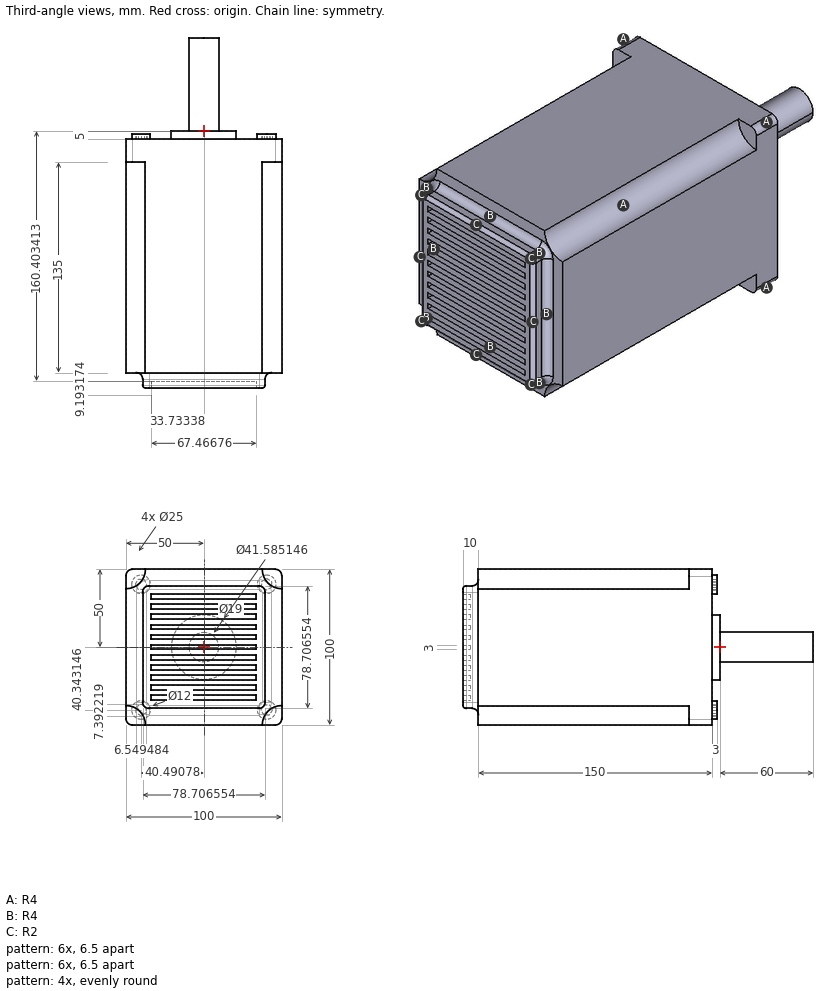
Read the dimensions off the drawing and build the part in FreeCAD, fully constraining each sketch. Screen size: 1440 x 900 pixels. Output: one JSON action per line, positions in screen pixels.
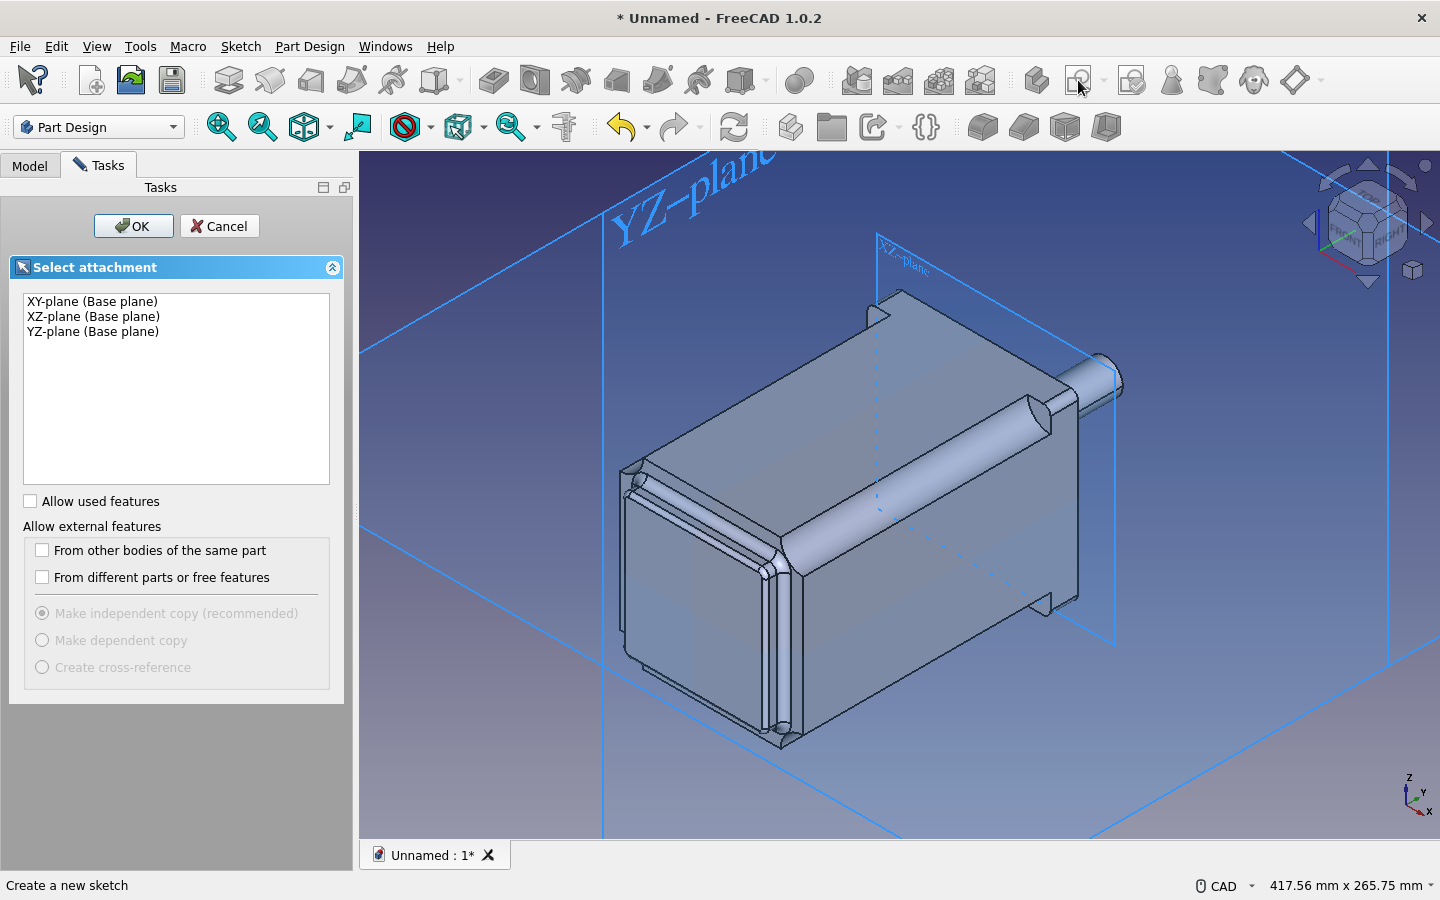
{"action": "left_click", "coordinate": [84, 302]}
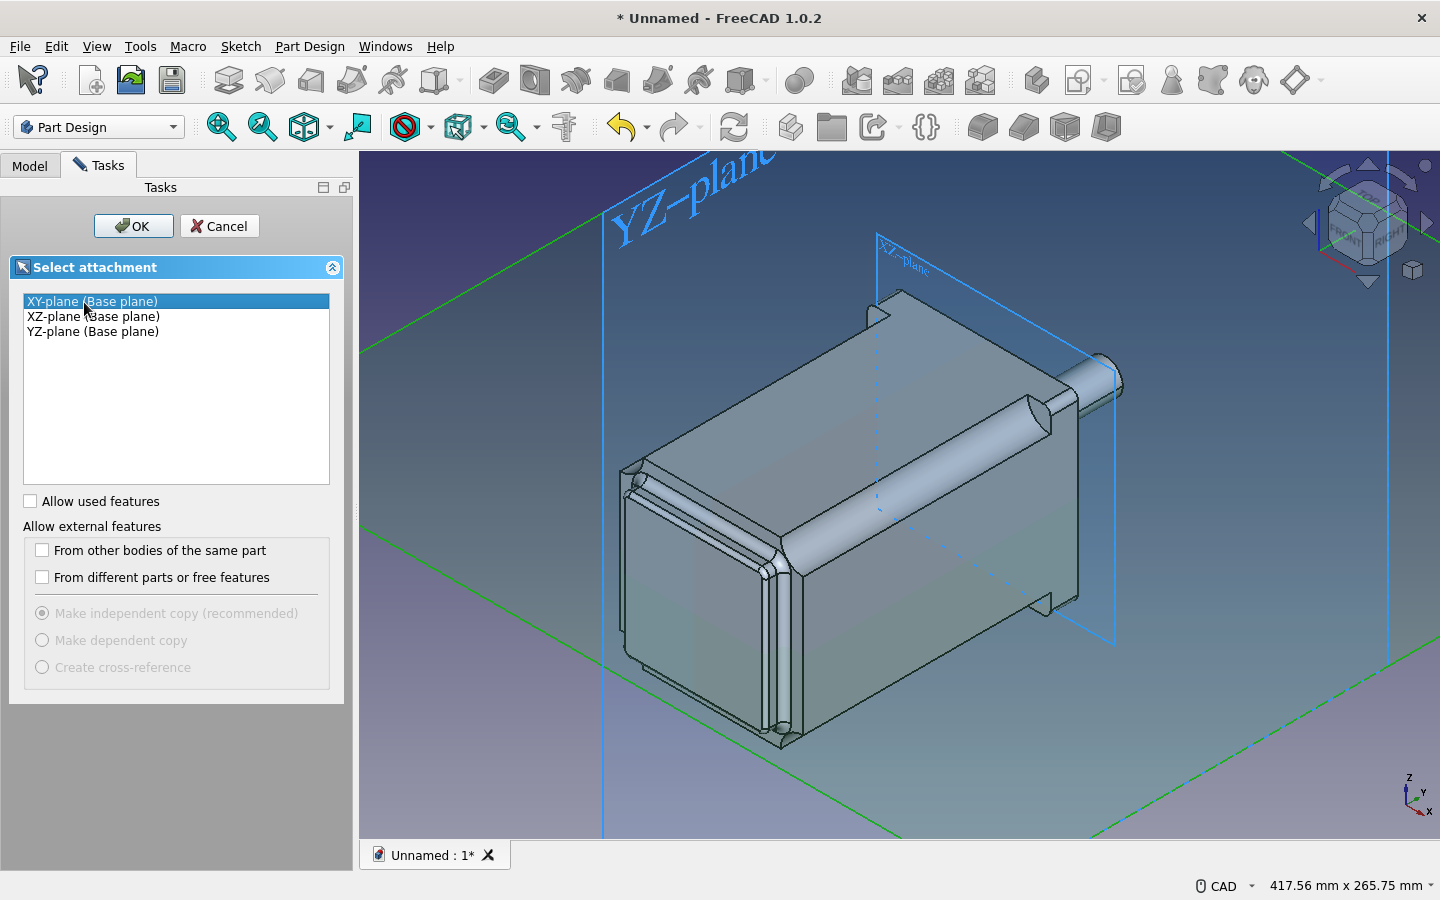
{"action": "left_click", "coordinate": [134, 226]}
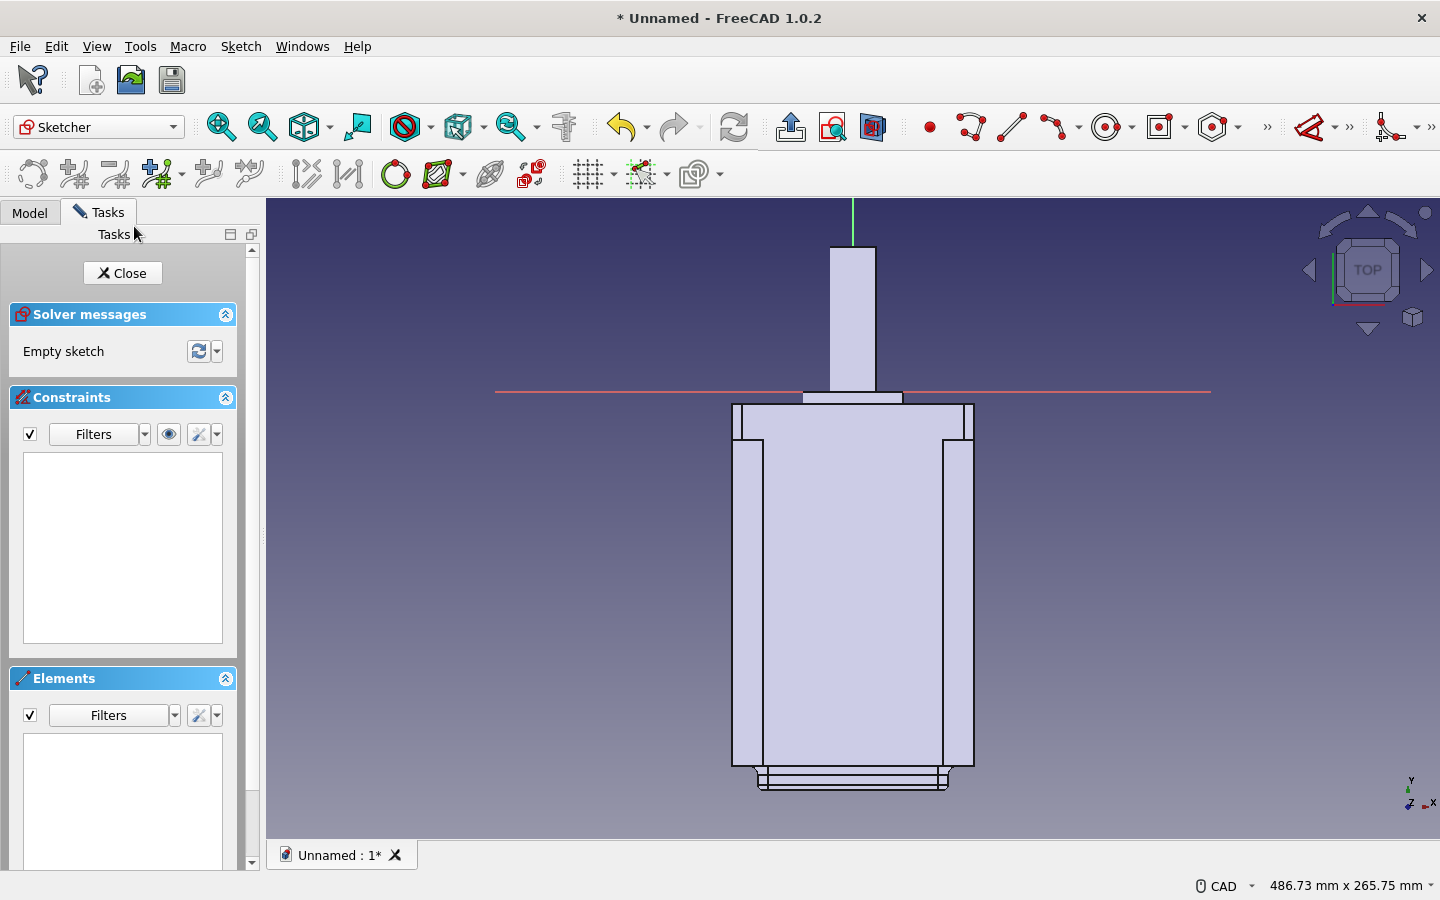
{"action": "left_click", "coordinate": [873, 128]}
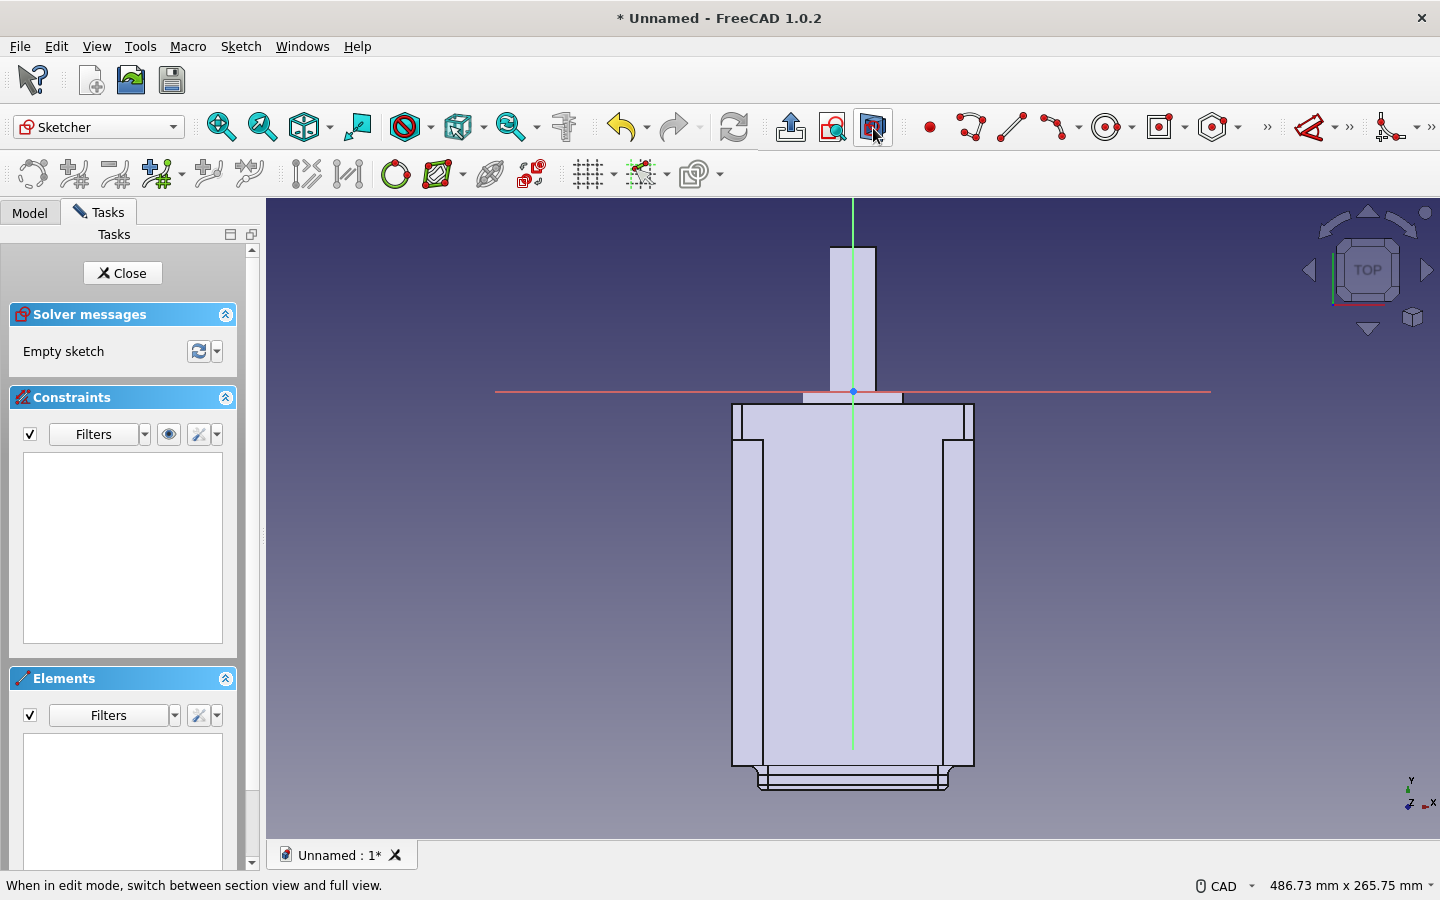
{"action": "scroll", "coordinate": [875, 811], "scroll_direction": "up", "scroll_amount": 7}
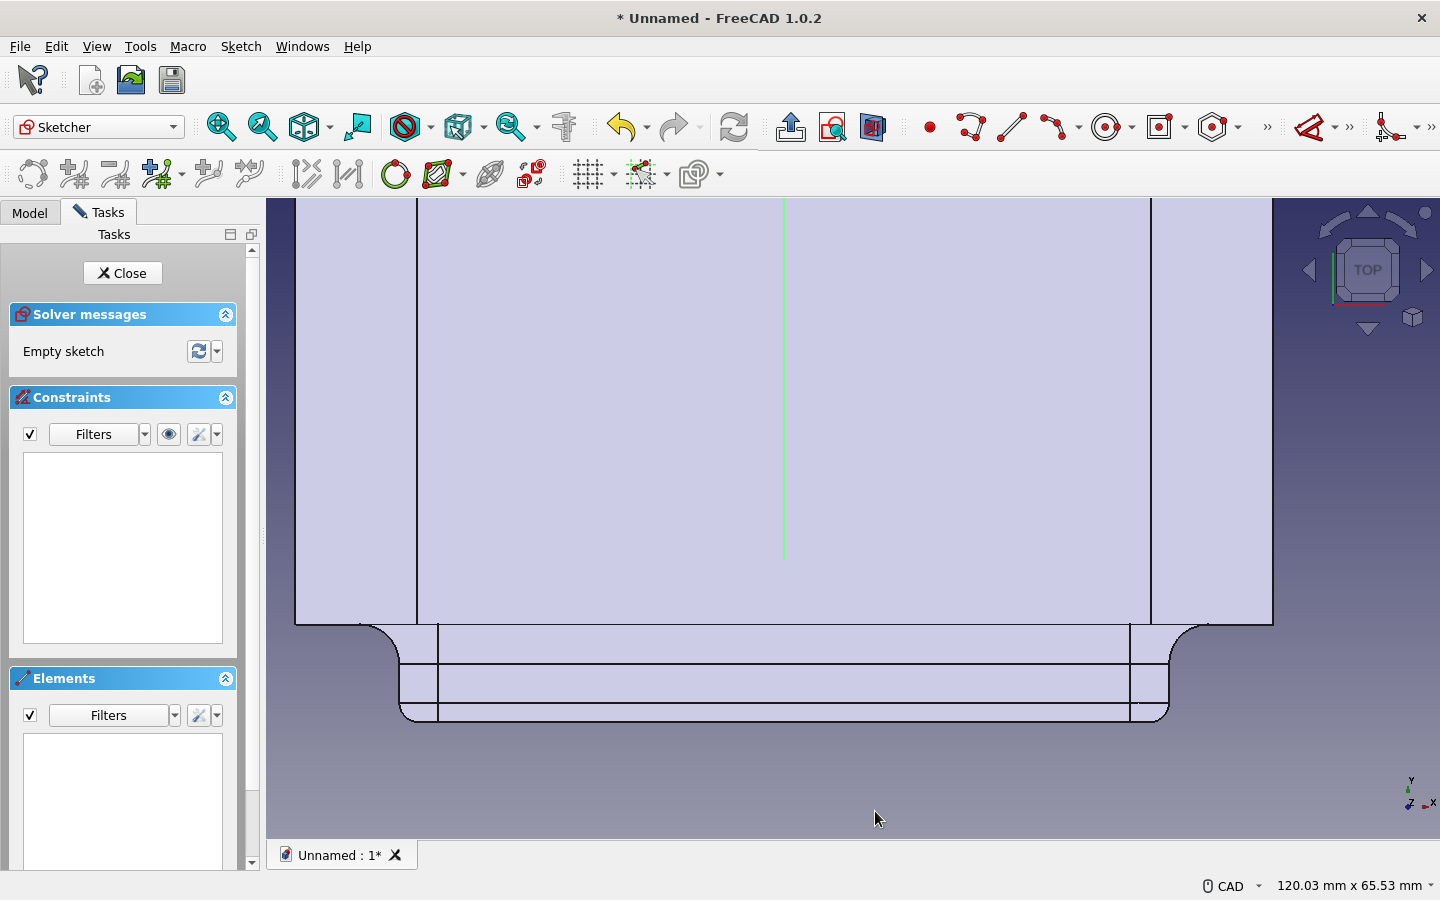
{"action": "left_click", "coordinate": [1184, 128]}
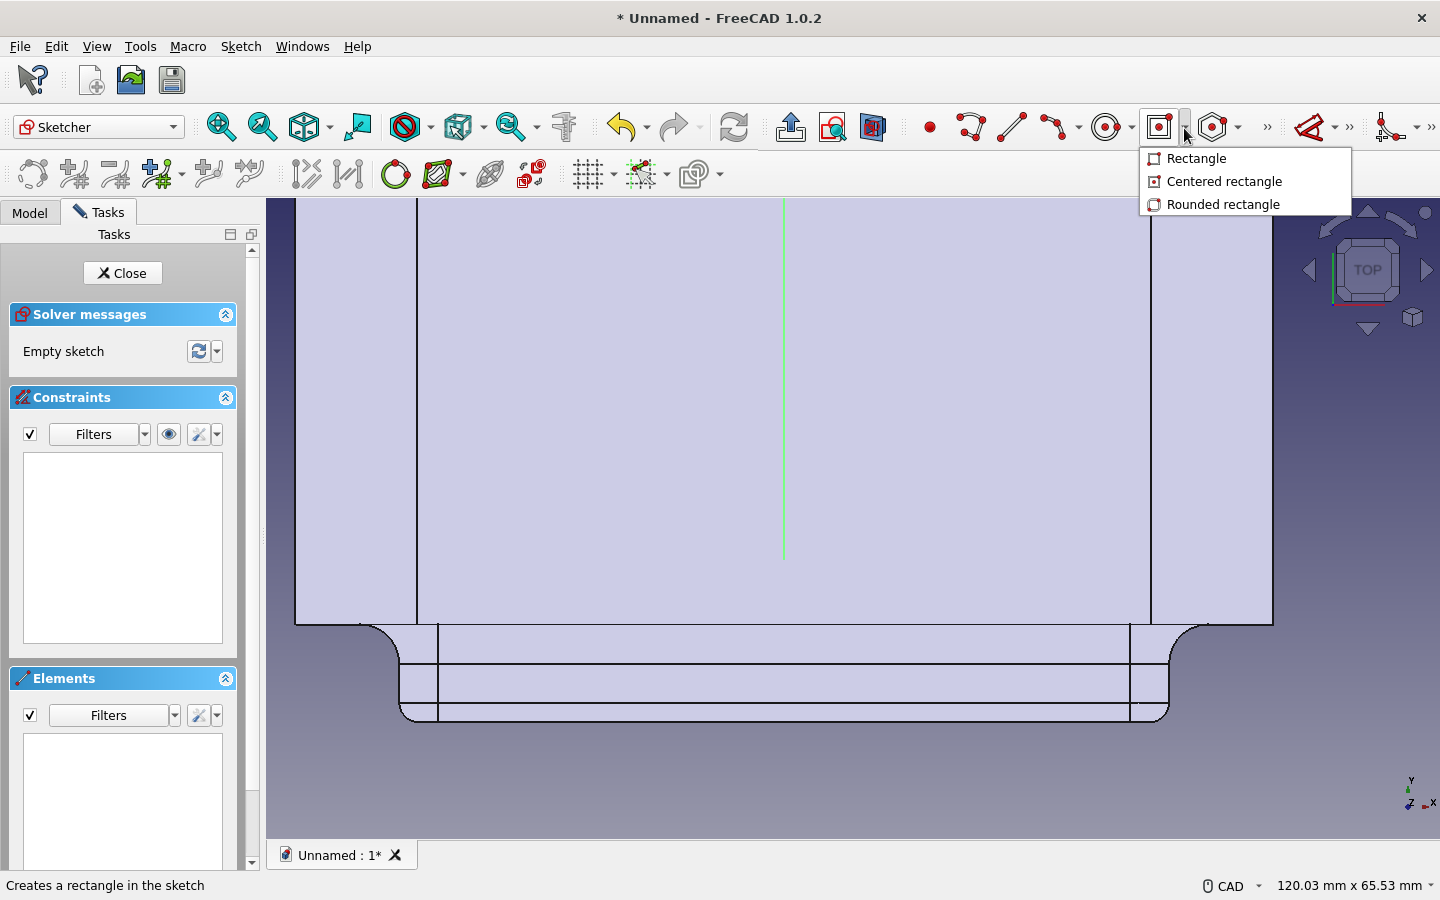
{"action": "left_click", "coordinate": [1246, 158]}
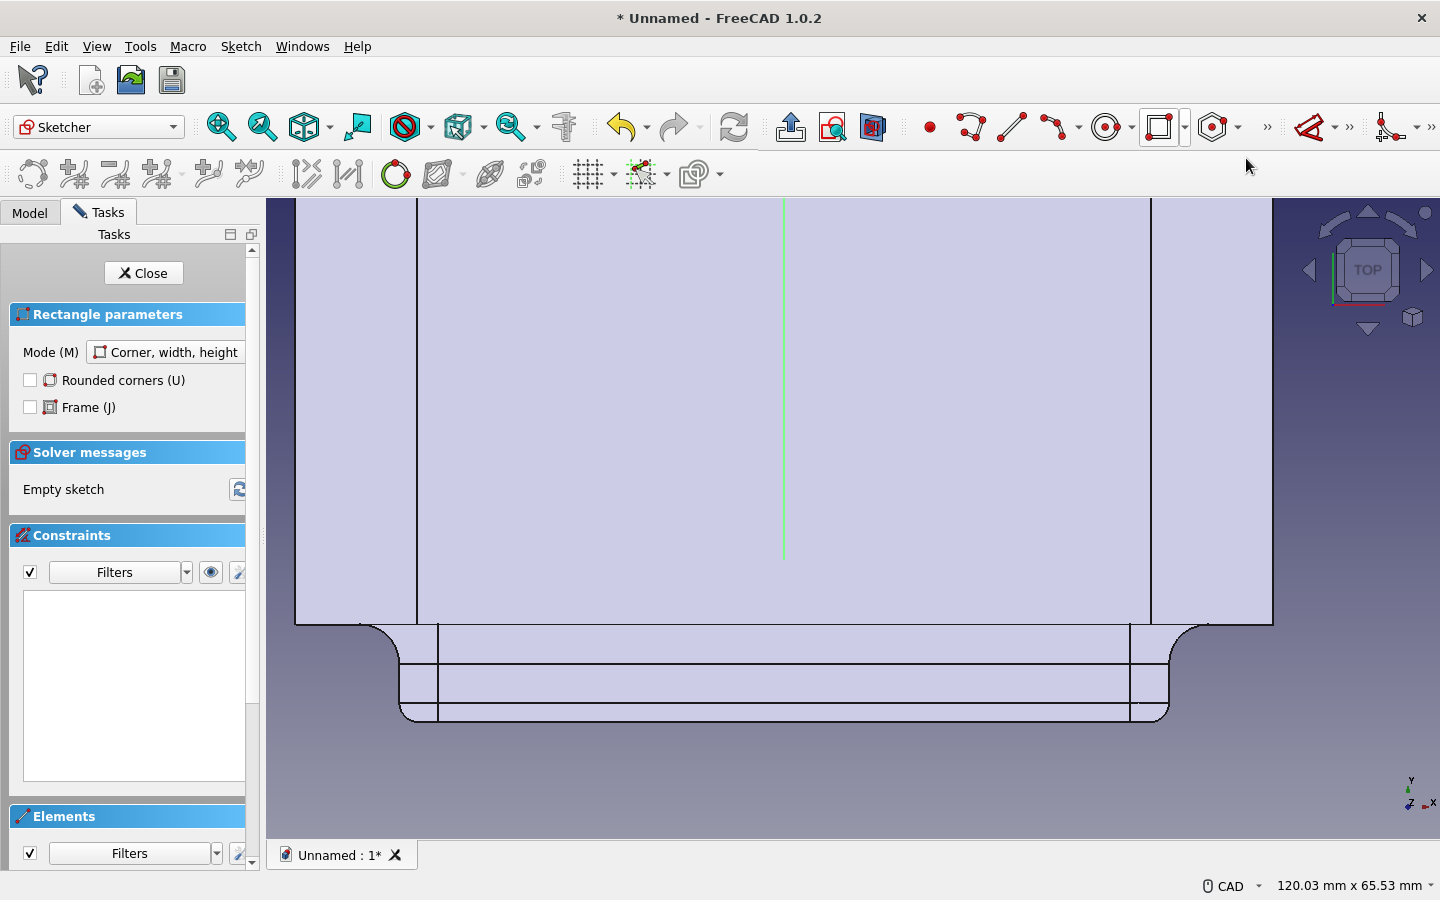
{"action": "left_click", "coordinate": [454, 677]}
{"action": "left_click", "coordinate": [1114, 767]}
{"action": "key", "text": "Escape"}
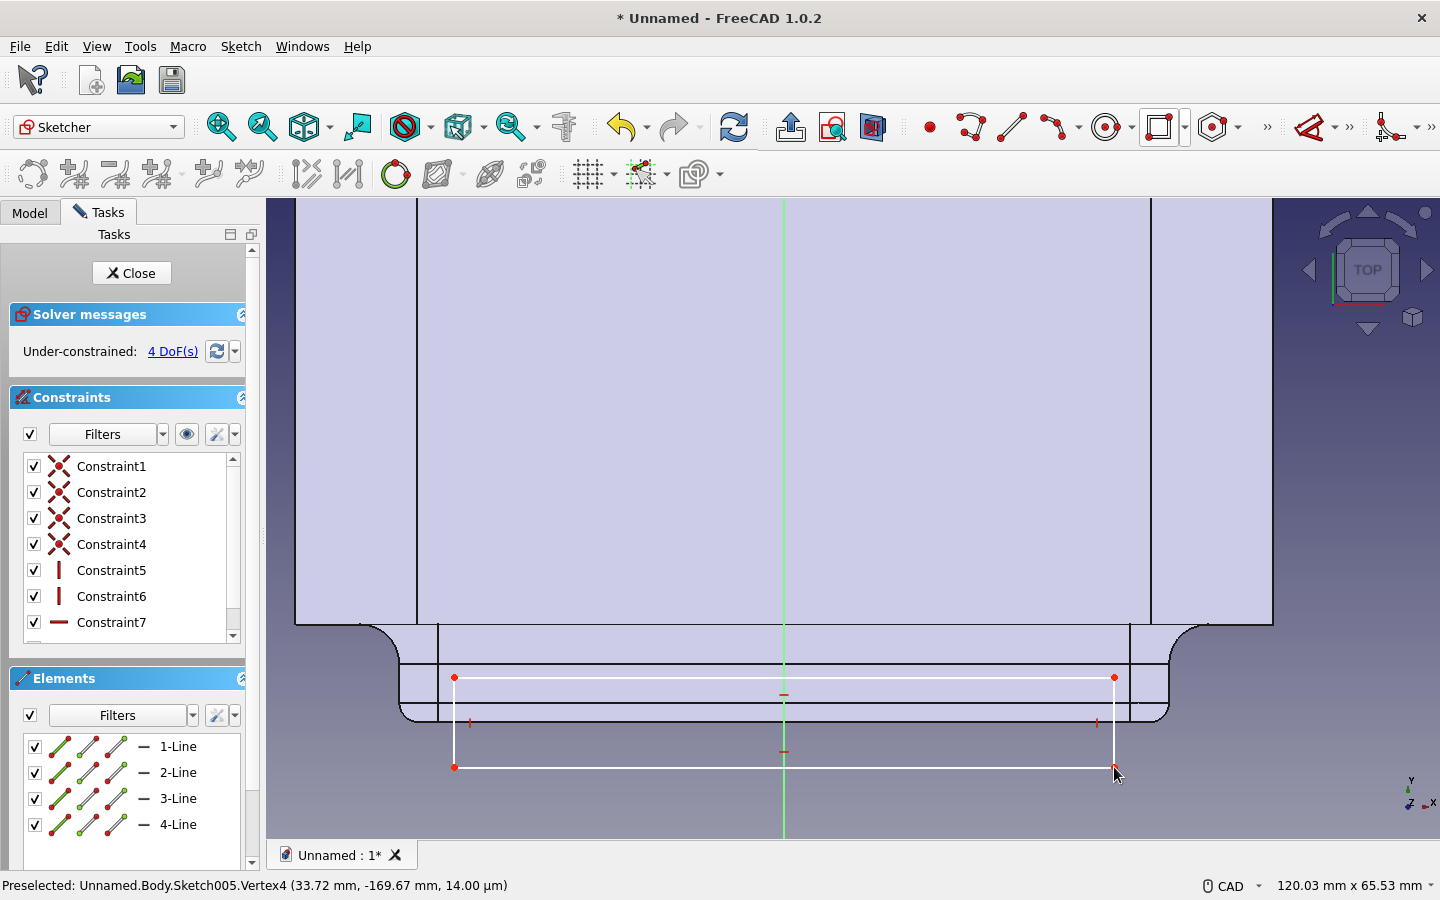
{"action": "key", "text": "d"}